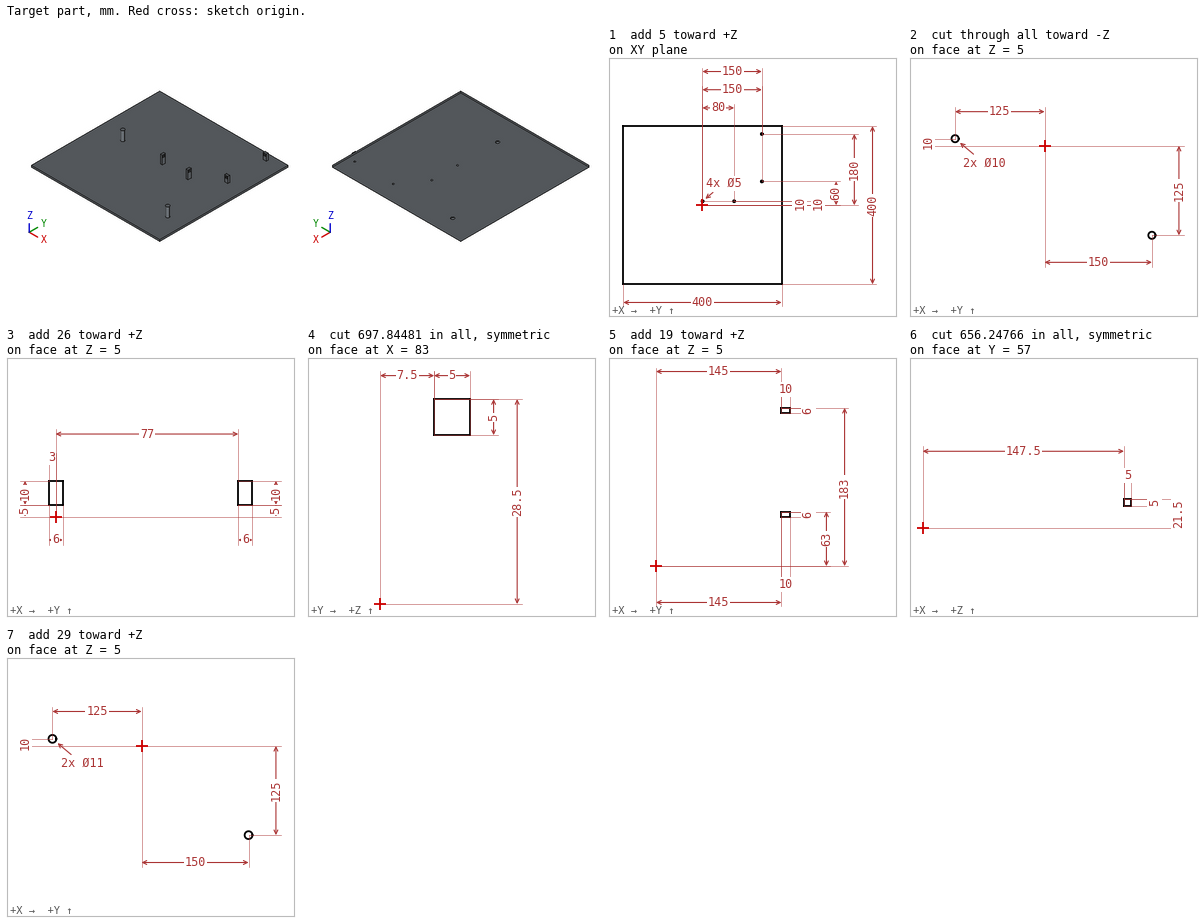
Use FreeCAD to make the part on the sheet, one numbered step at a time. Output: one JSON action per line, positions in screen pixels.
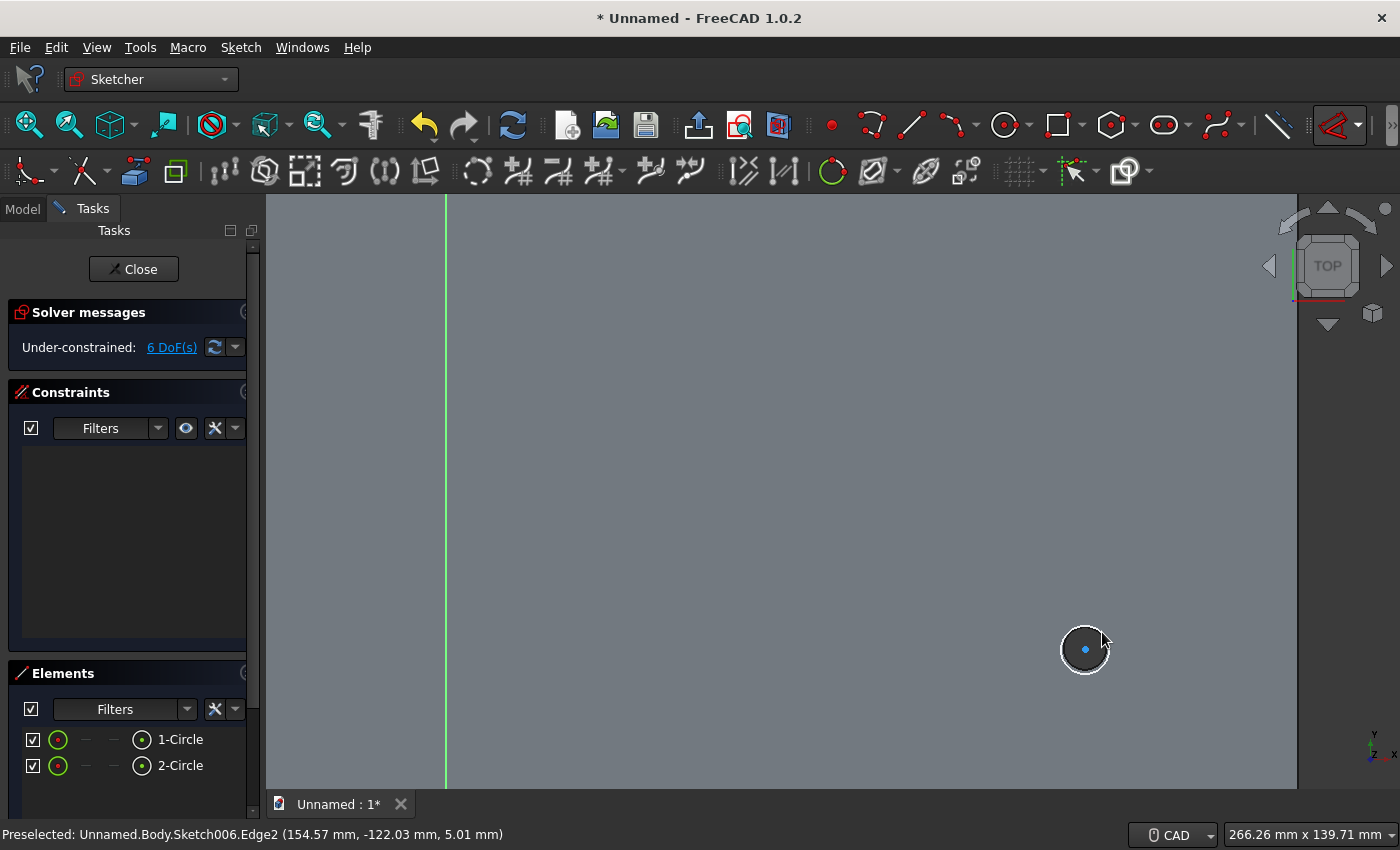
{"action": "scroll", "coordinate": [1087, 650], "scroll_direction": "down", "scroll_amount": 3}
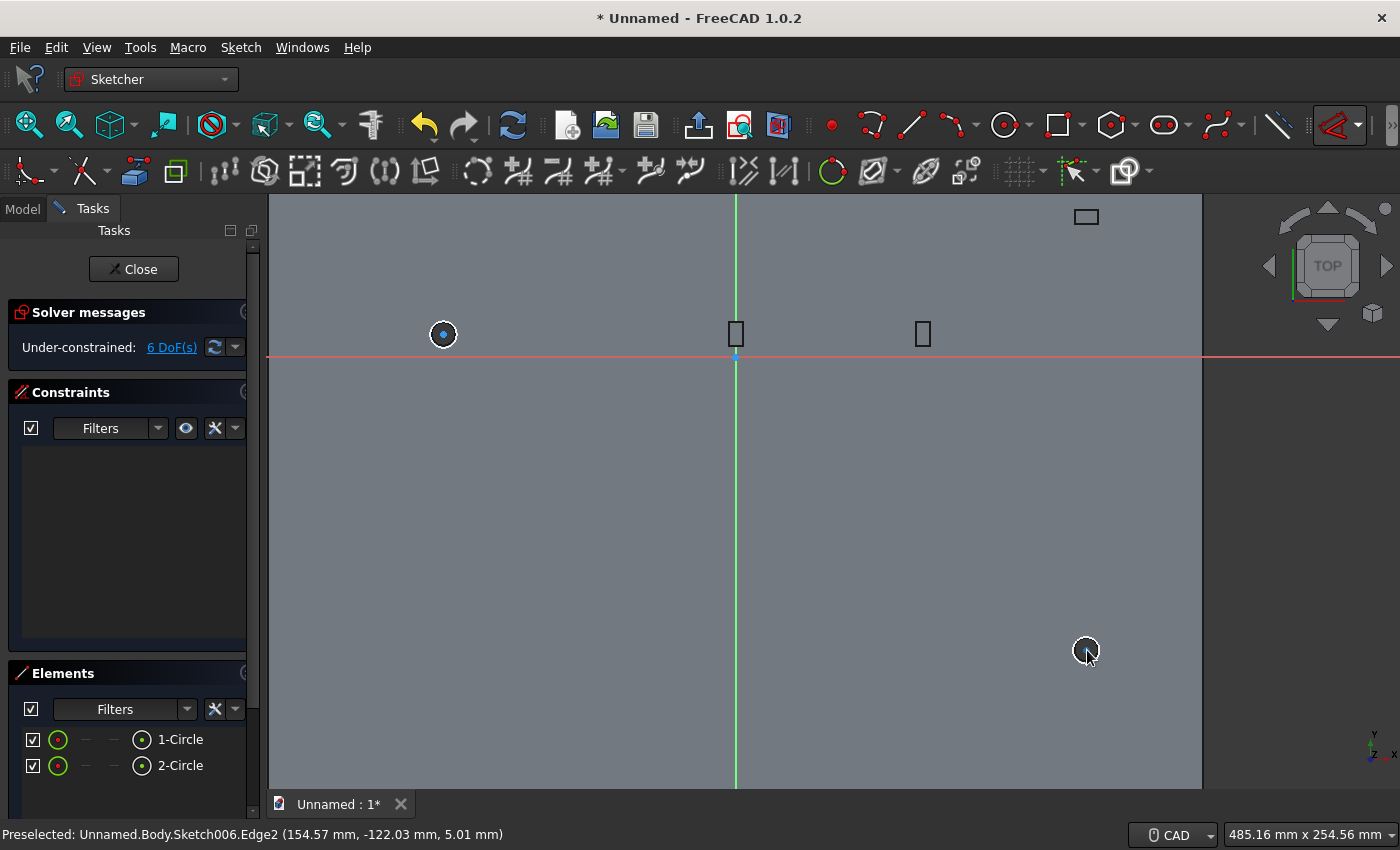
{"action": "left_click", "coordinate": [453, 325]}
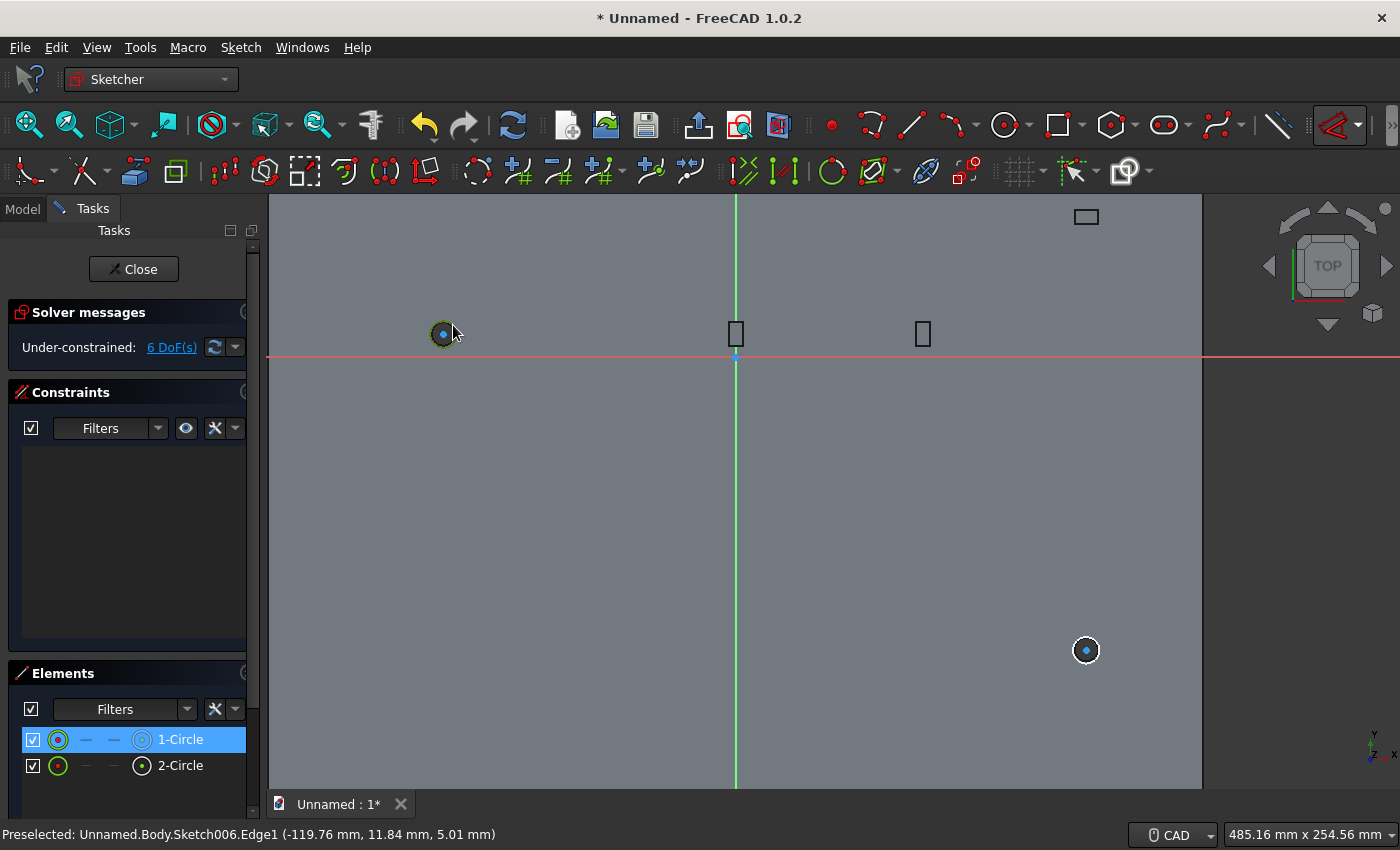
{"action": "left_click", "coordinate": [1096, 641]}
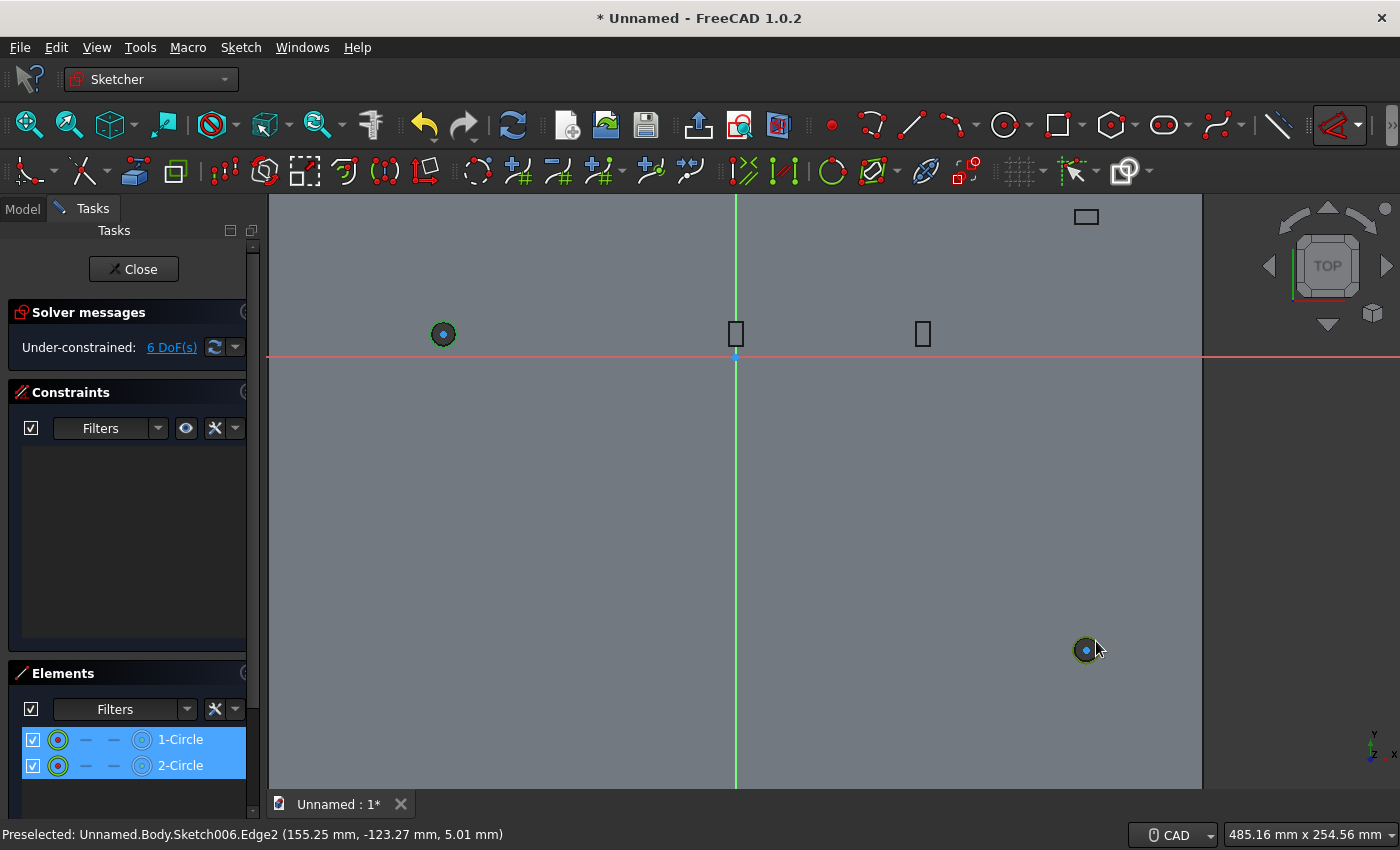
{"action": "key", "text": "e"}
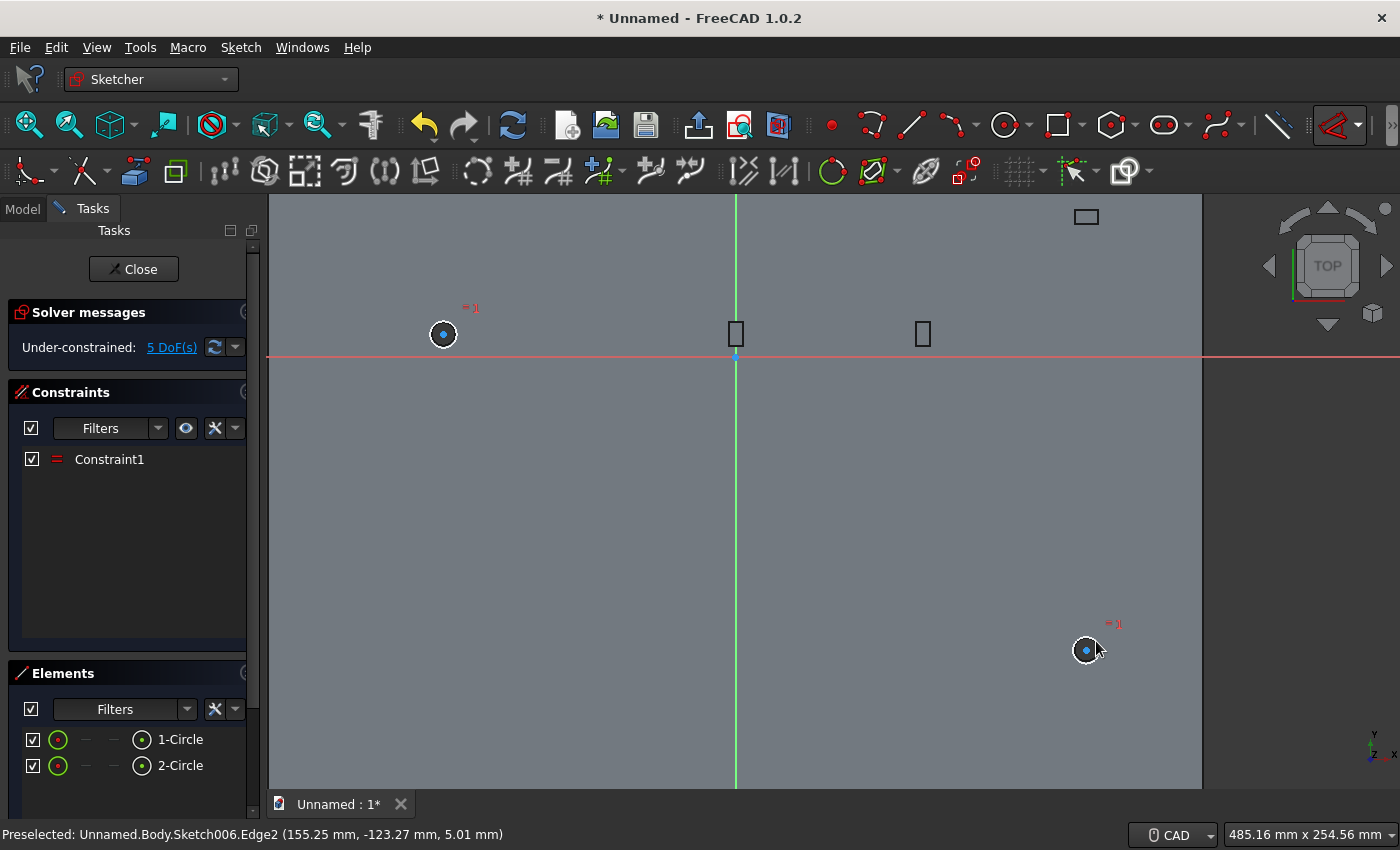
{"action": "scroll", "coordinate": [453, 325], "scroll_direction": "up", "scroll_amount": 3}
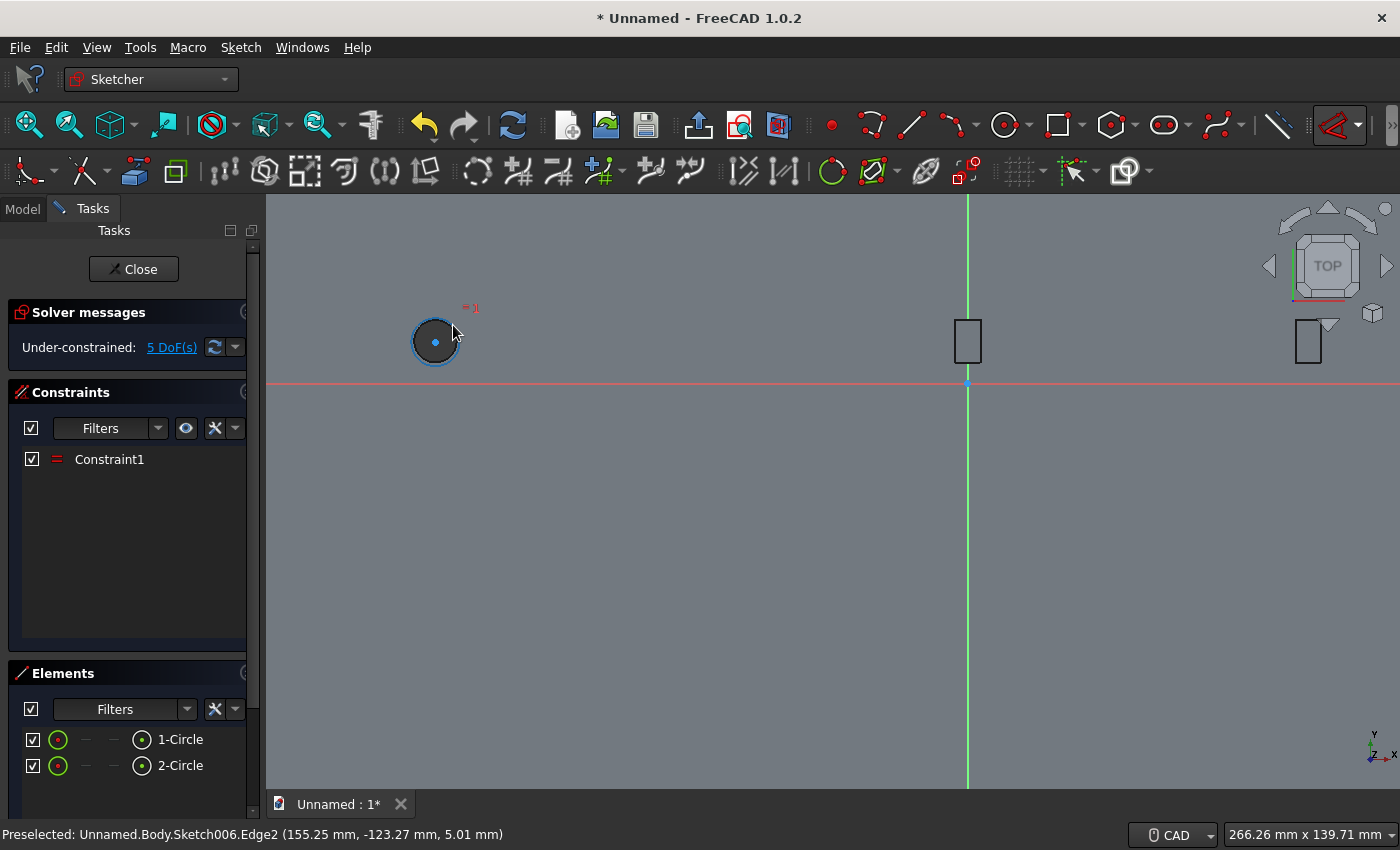
{"action": "left_click", "coordinate": [452, 325]}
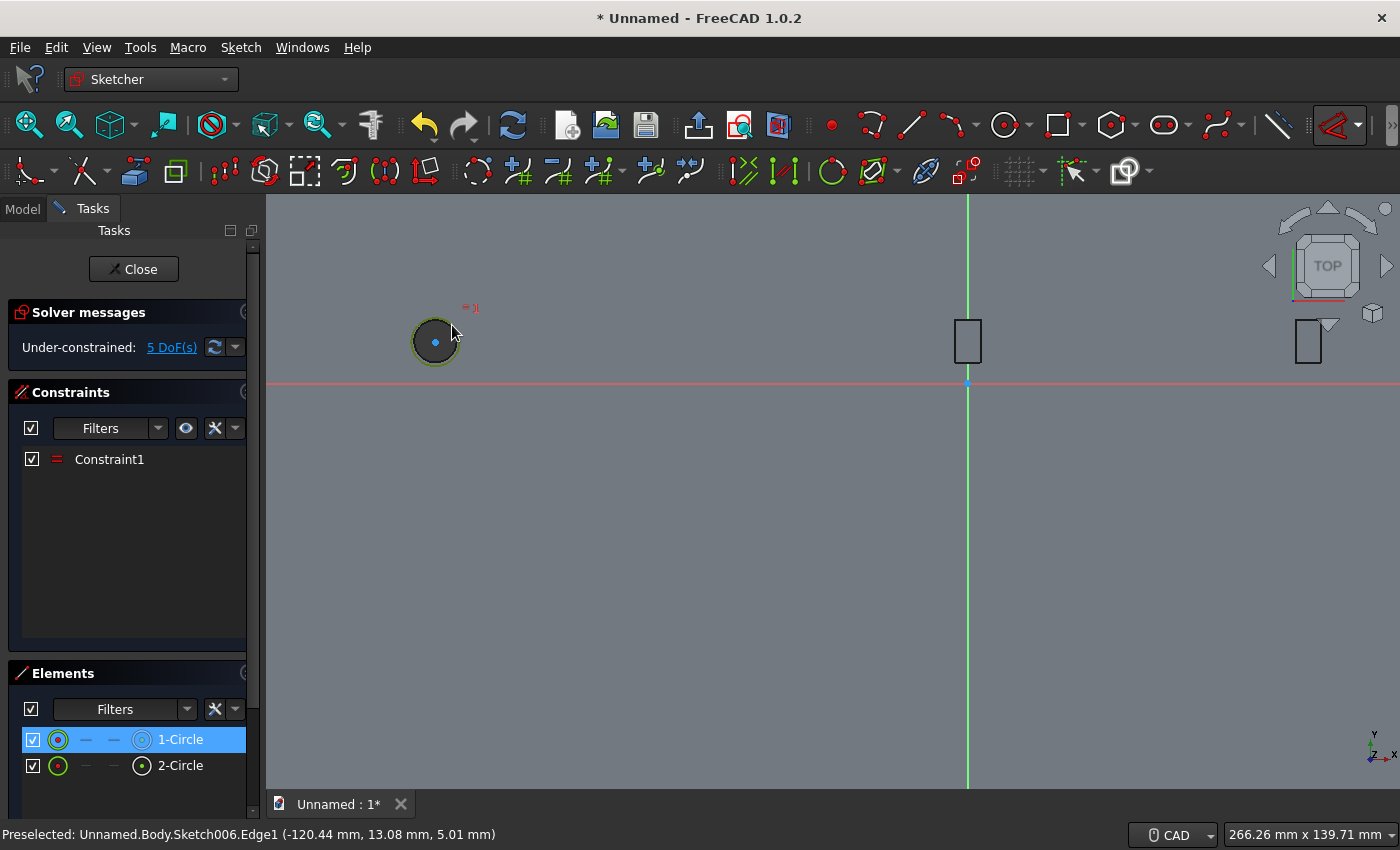
{"action": "key", "text": "k o"}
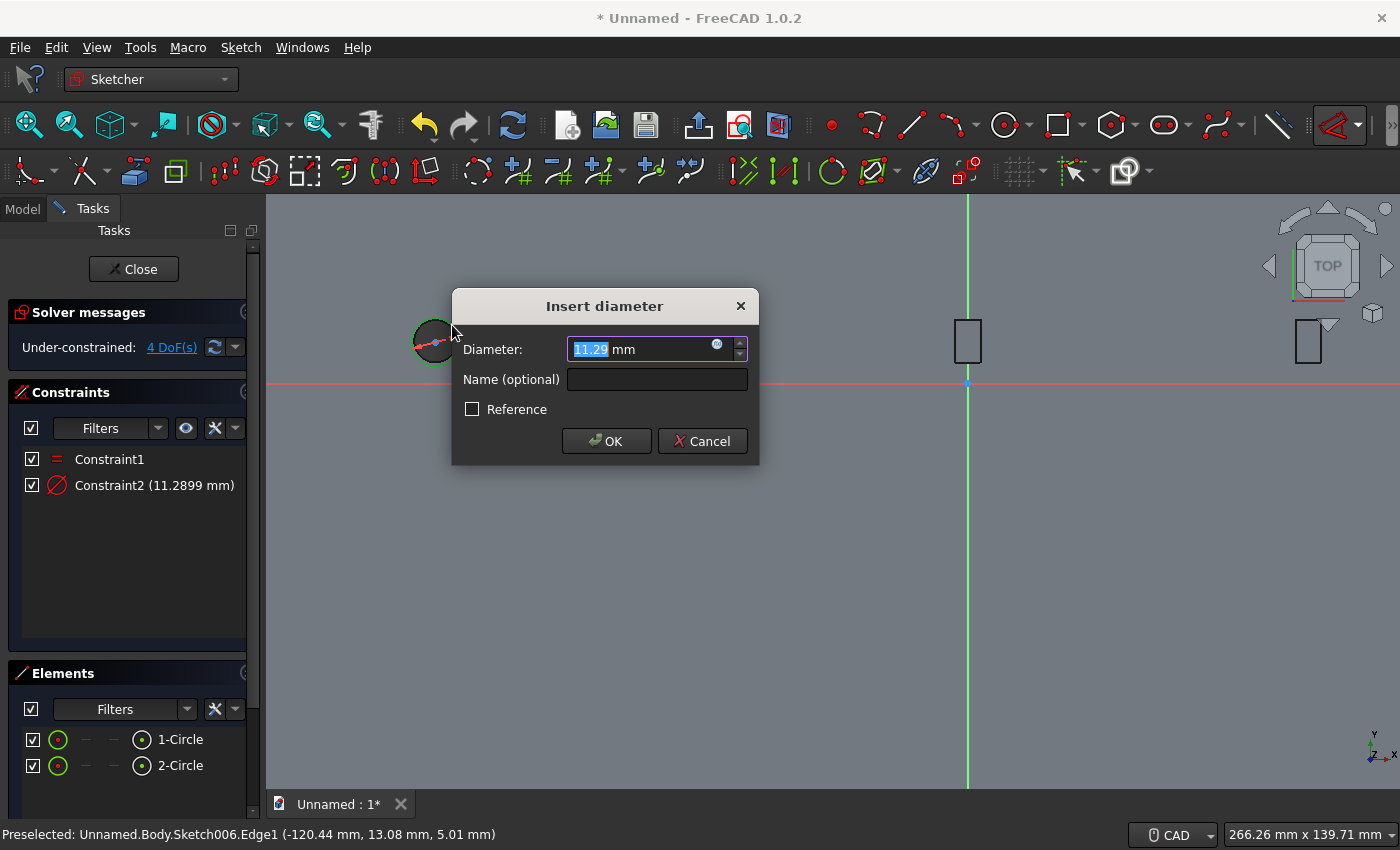
{"action": "type", "text": "11"}
{"action": "key", "text": "Return"}